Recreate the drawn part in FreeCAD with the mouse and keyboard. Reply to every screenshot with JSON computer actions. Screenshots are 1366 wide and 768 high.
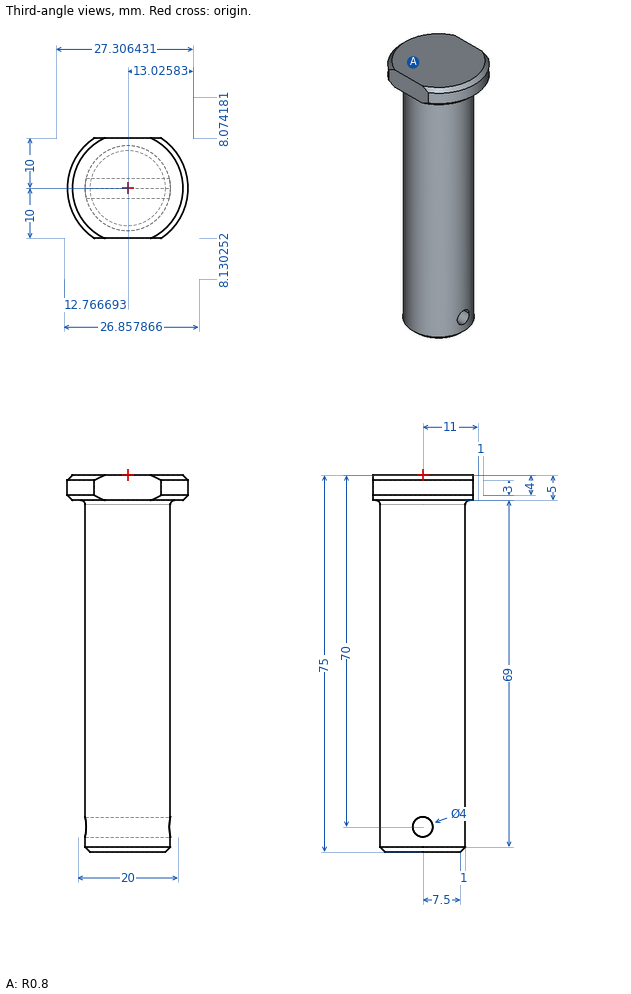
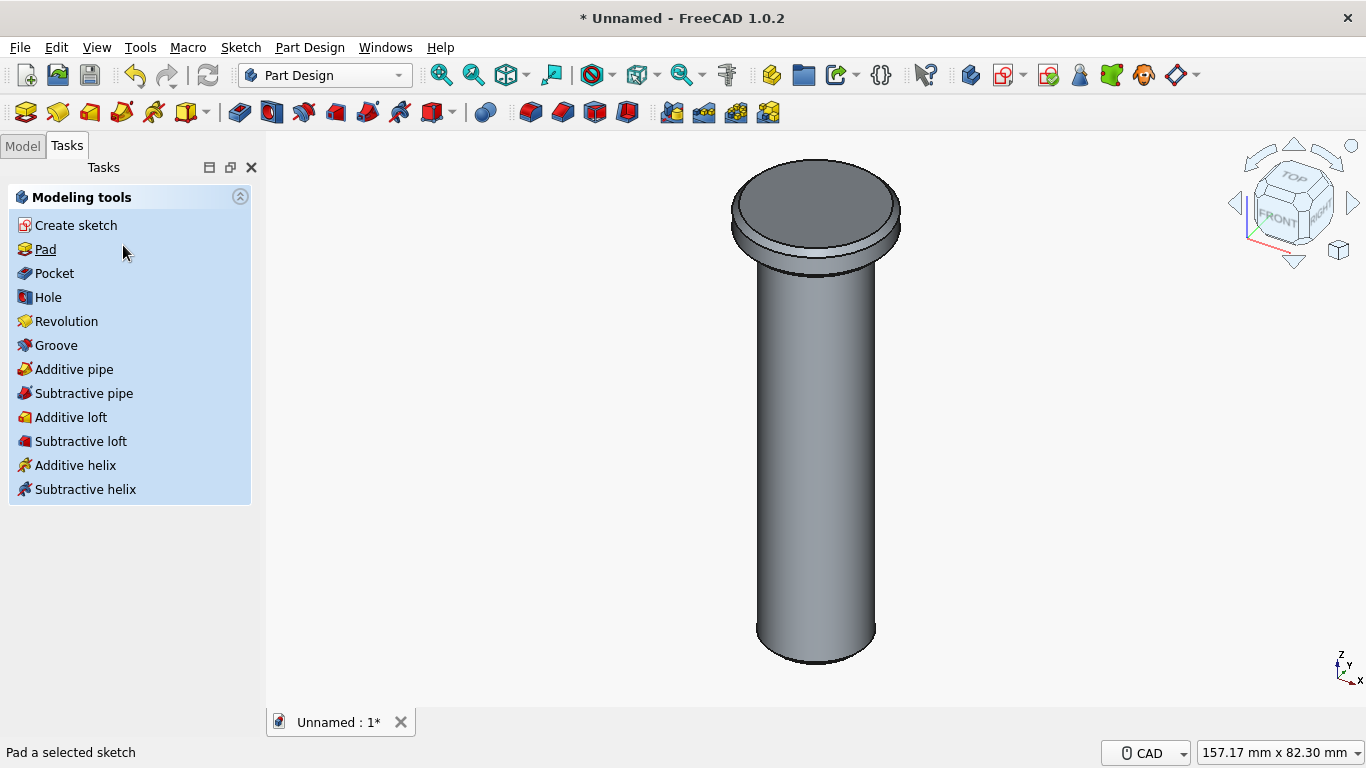
{"action": "left_click", "coordinate": [240, 112]}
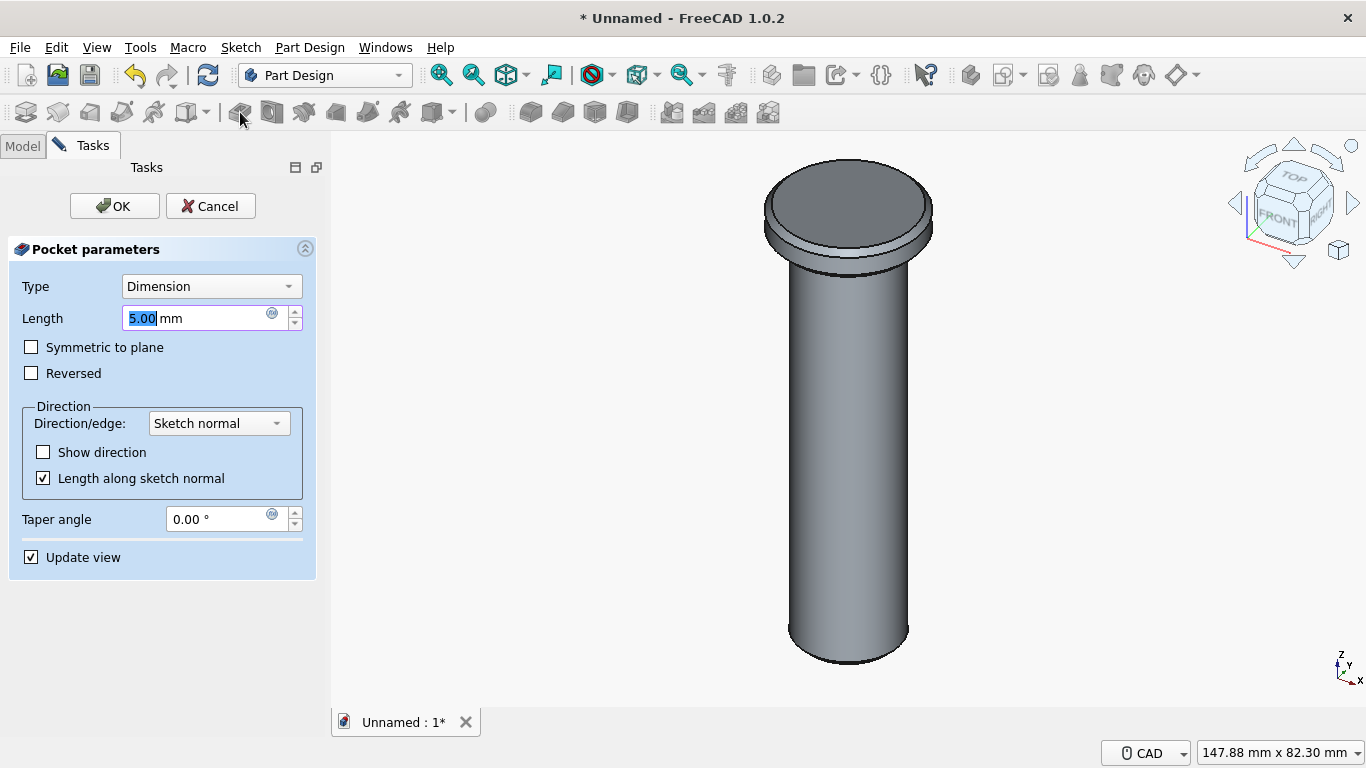
{"action": "type", "text": "20"}
{"action": "key", "text": "Tab"}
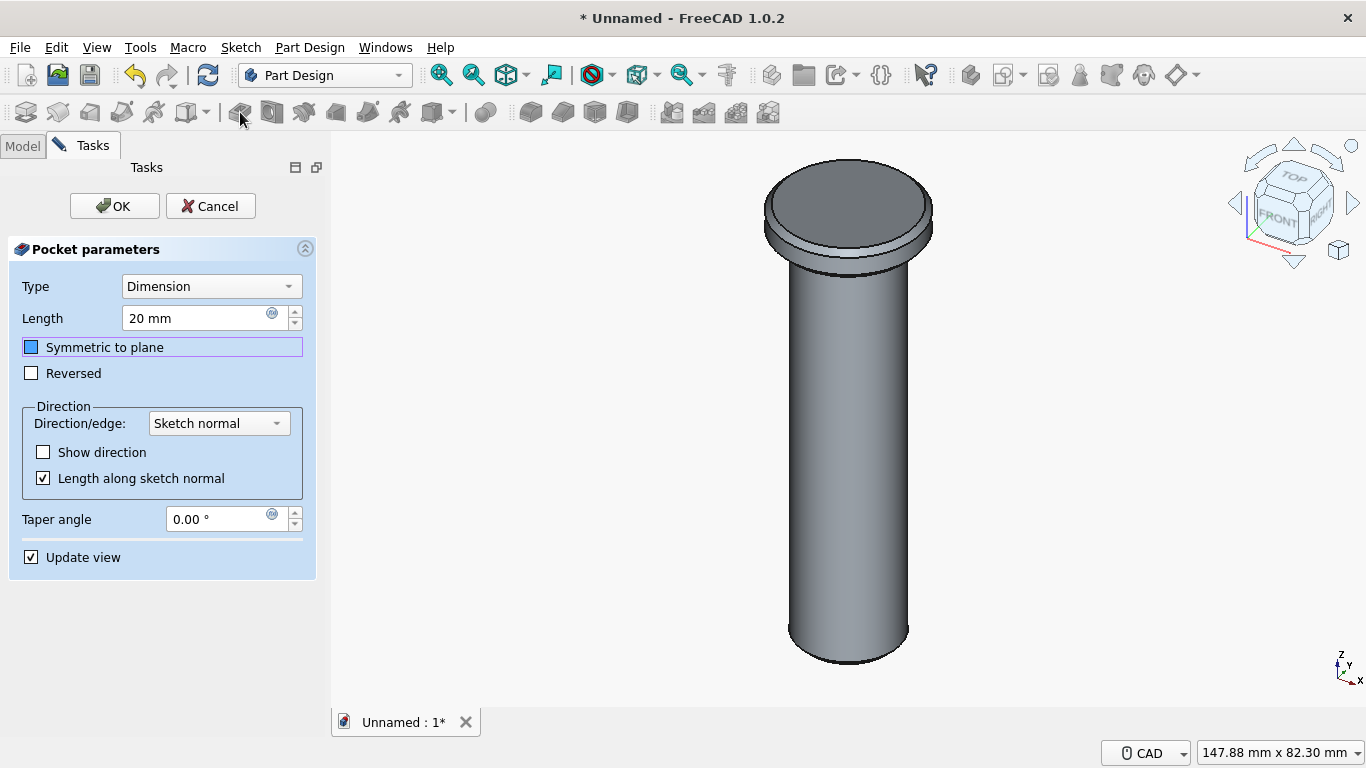
{"action": "left_click", "coordinate": [30, 347]}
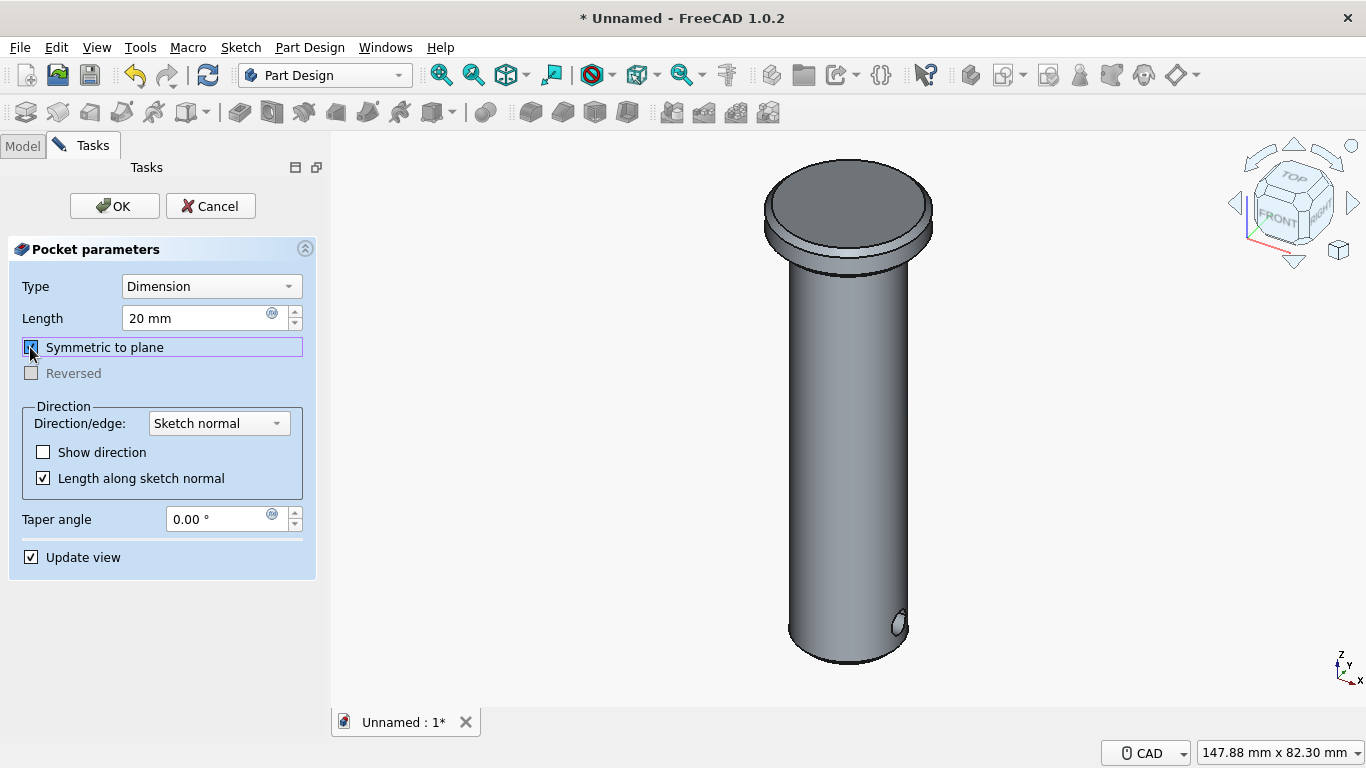
{"action": "left_click", "coordinate": [115, 206]}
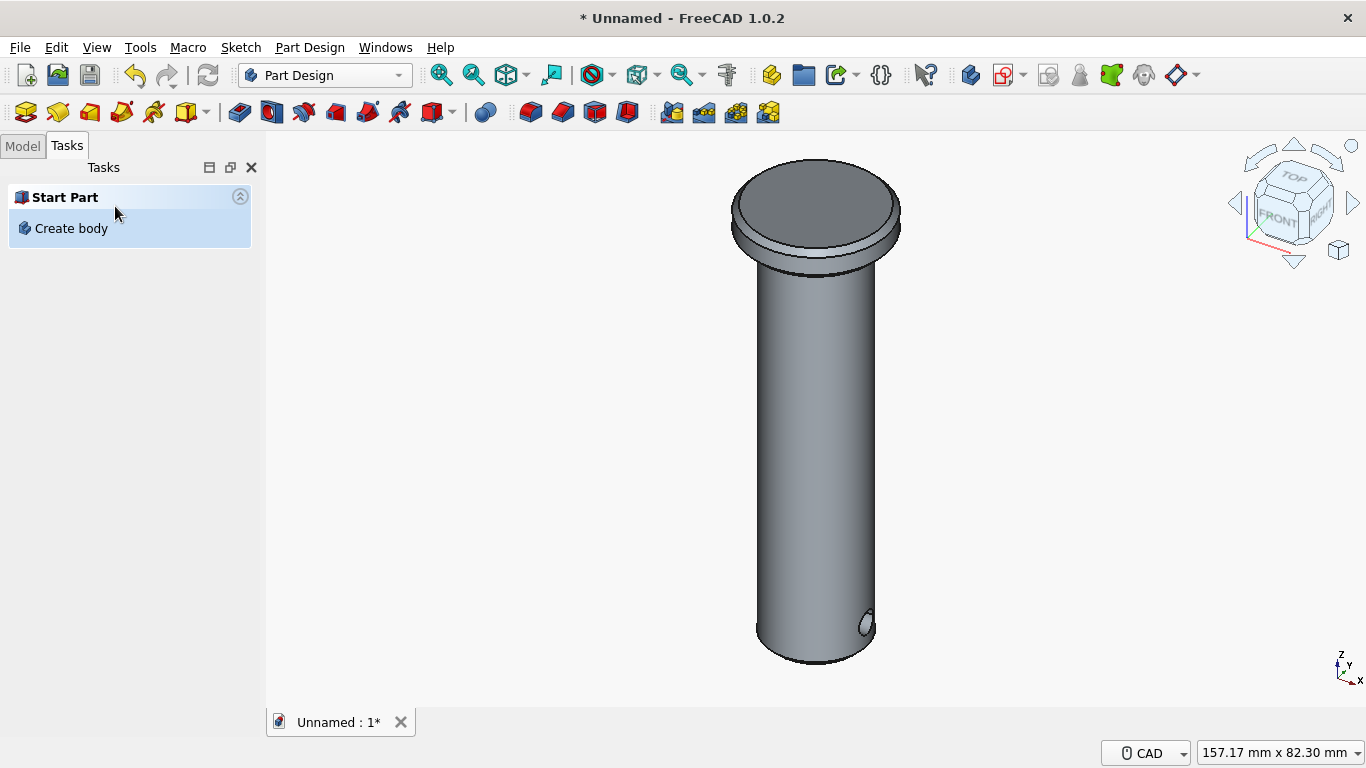
{"action": "left_click", "coordinate": [1004, 76]}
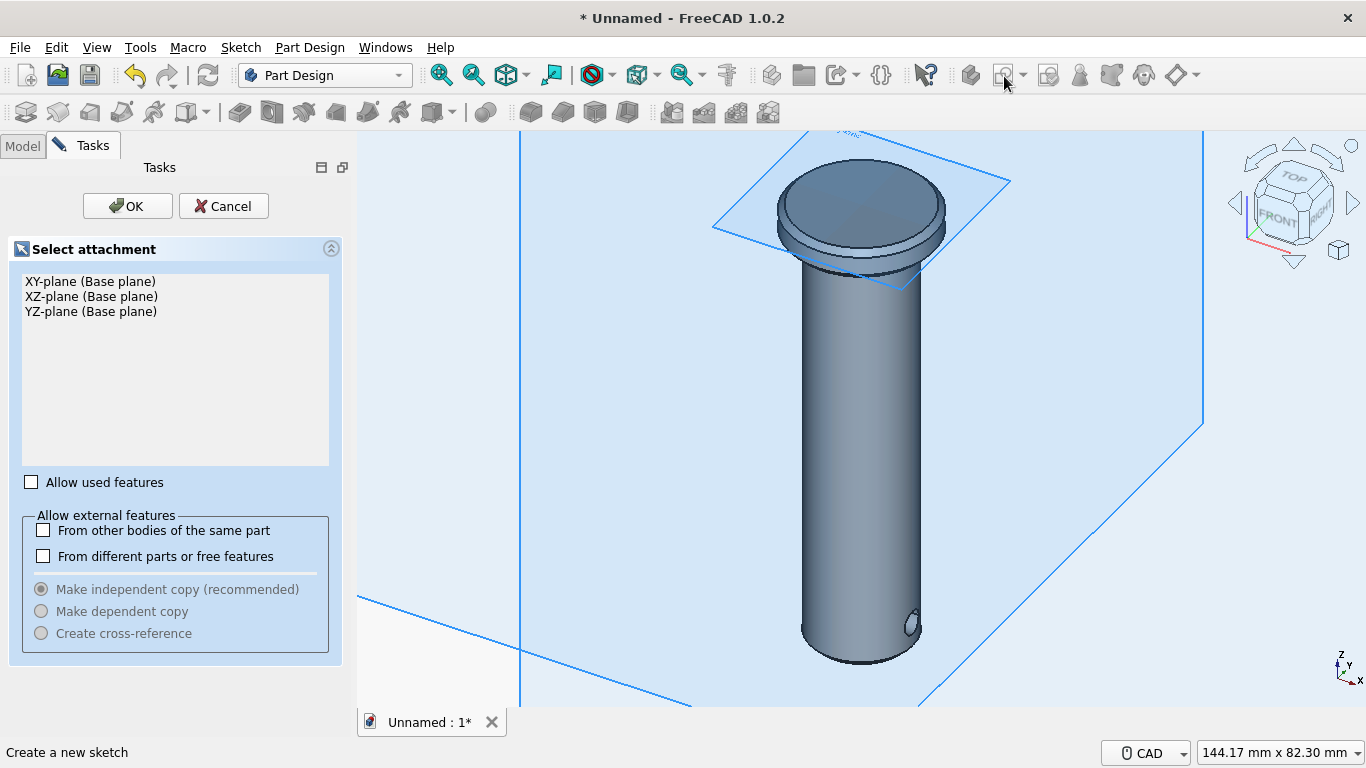
{"action": "left_click", "coordinate": [82, 282]}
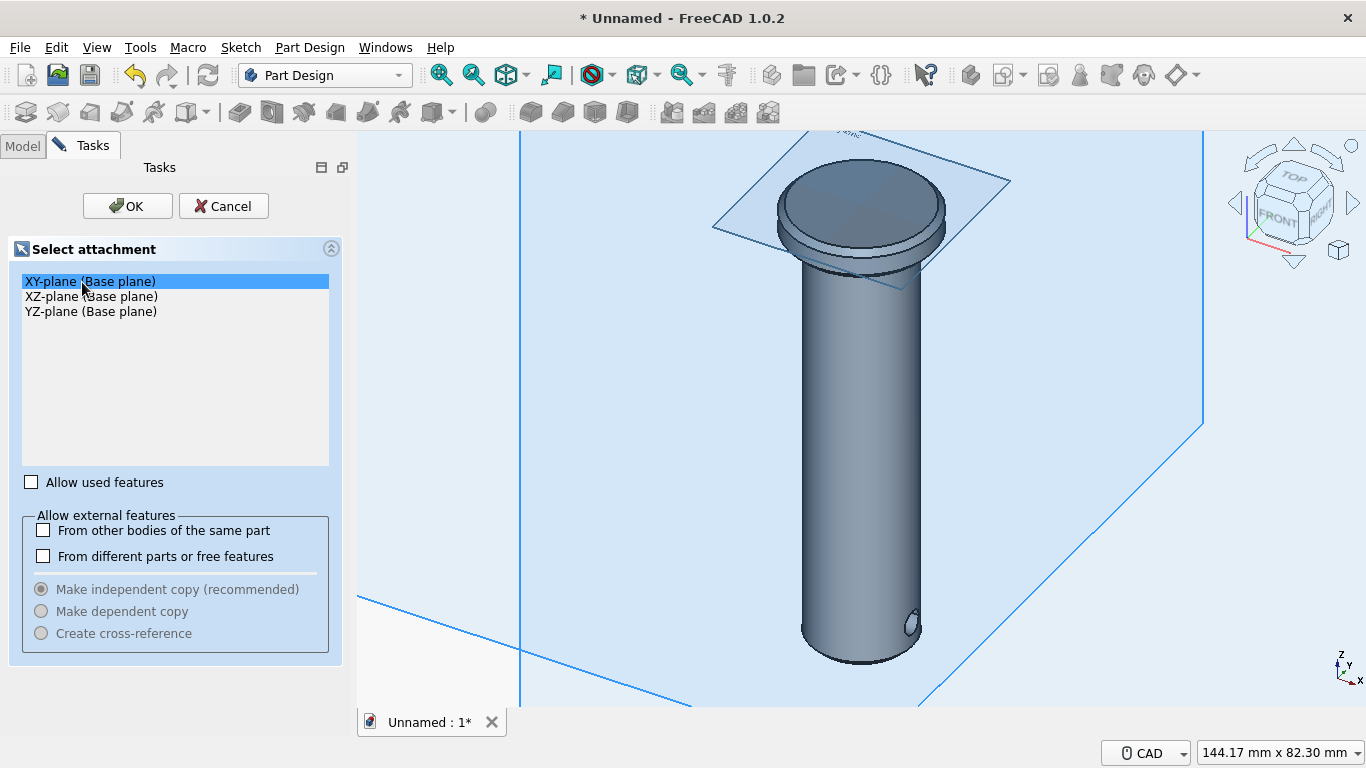
{"action": "left_click", "coordinate": [128, 206]}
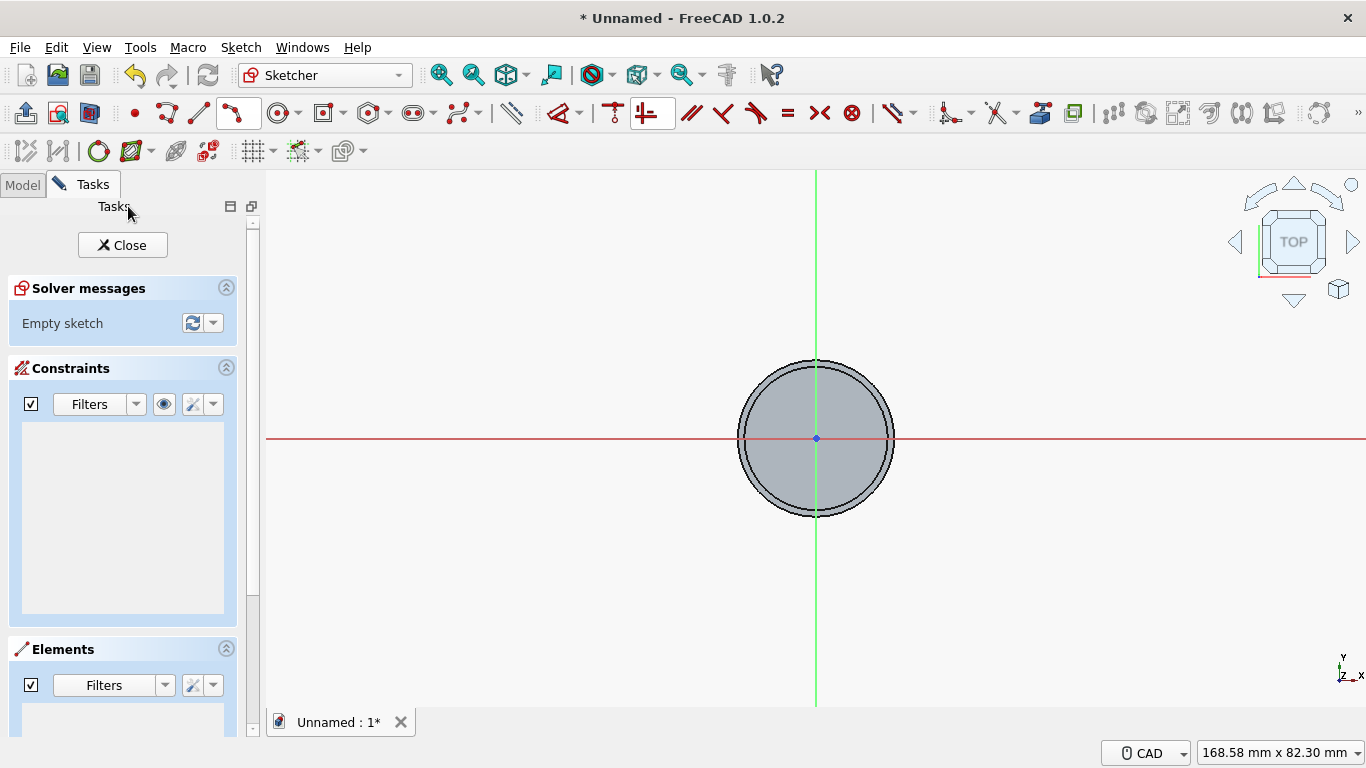
{"action": "scroll", "coordinate": [953, 439], "scroll_direction": "up", "scroll_amount": 2}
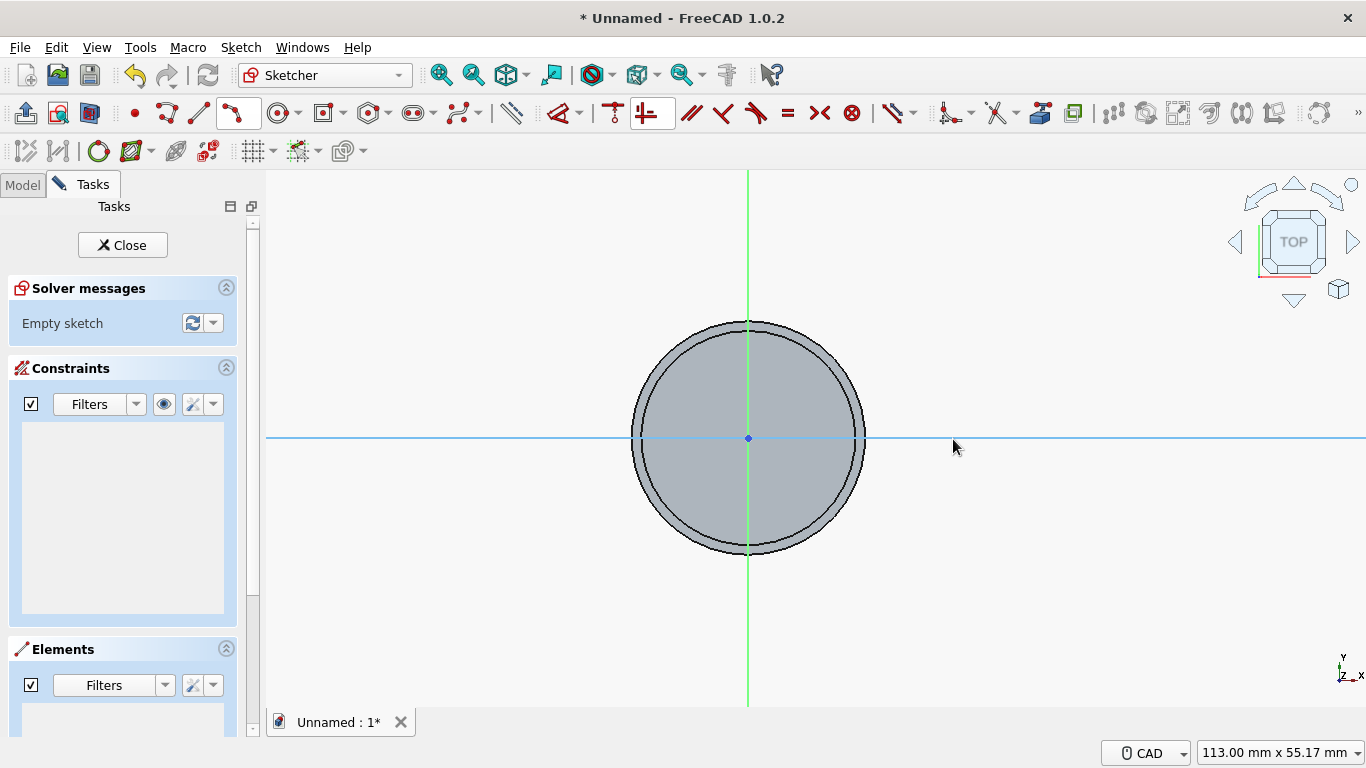
{"action": "left_click", "coordinate": [346, 114]}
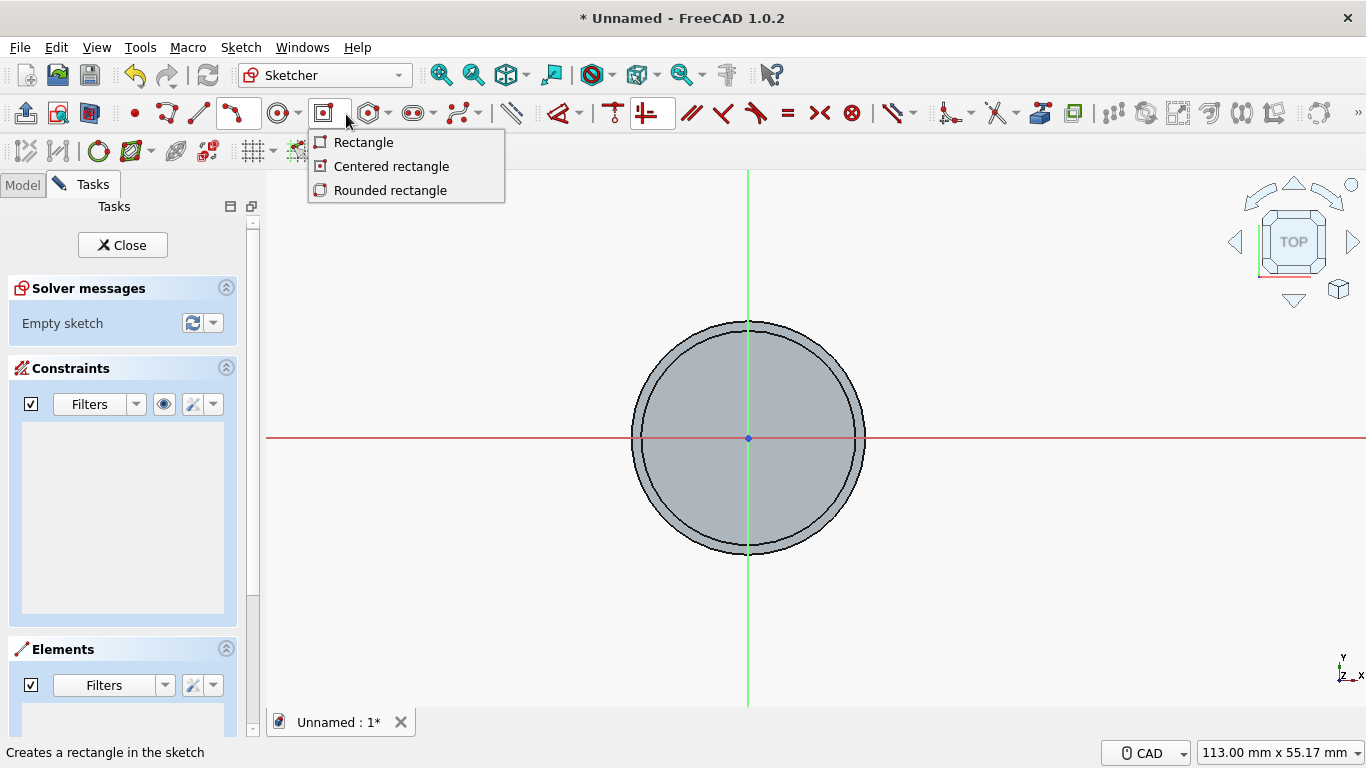
{"action": "left_click", "coordinate": [406, 142]}